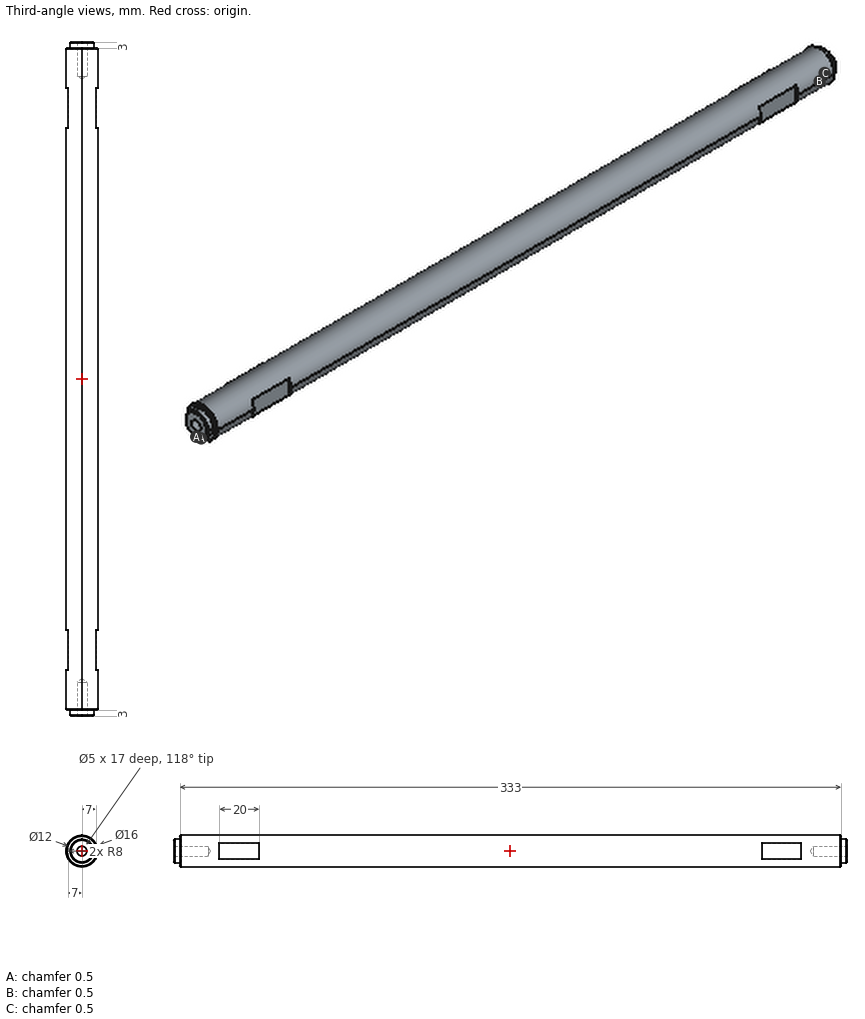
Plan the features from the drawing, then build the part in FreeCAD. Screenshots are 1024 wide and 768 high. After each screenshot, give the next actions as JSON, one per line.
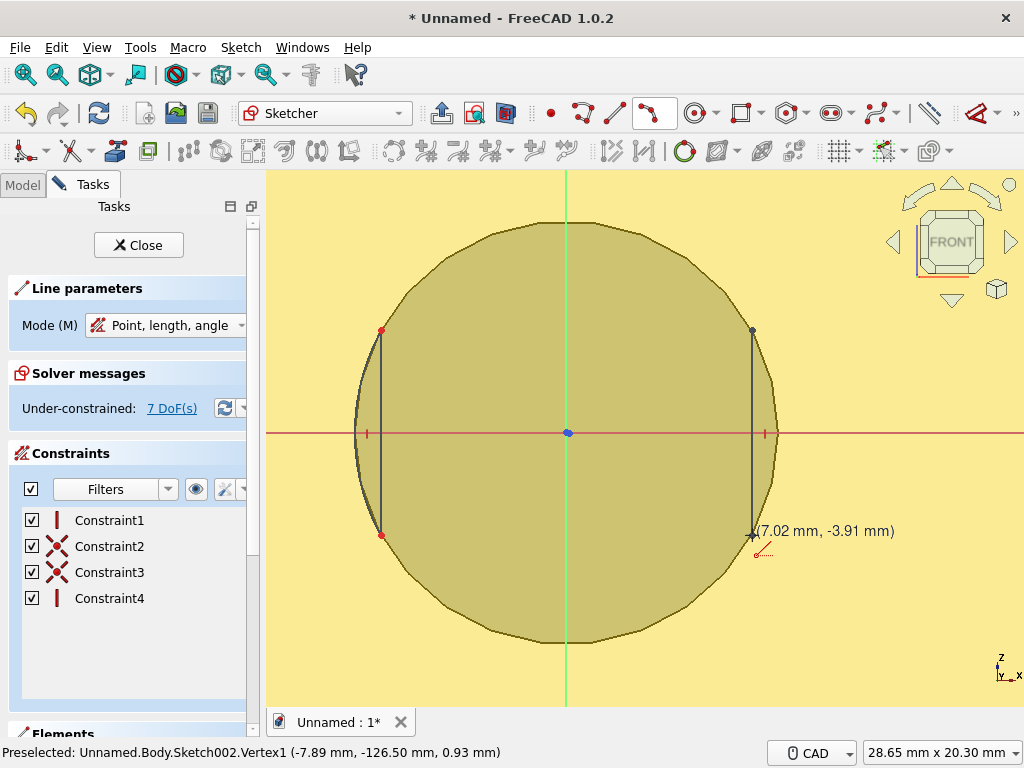
{"action": "key", "text": "g 3 a"}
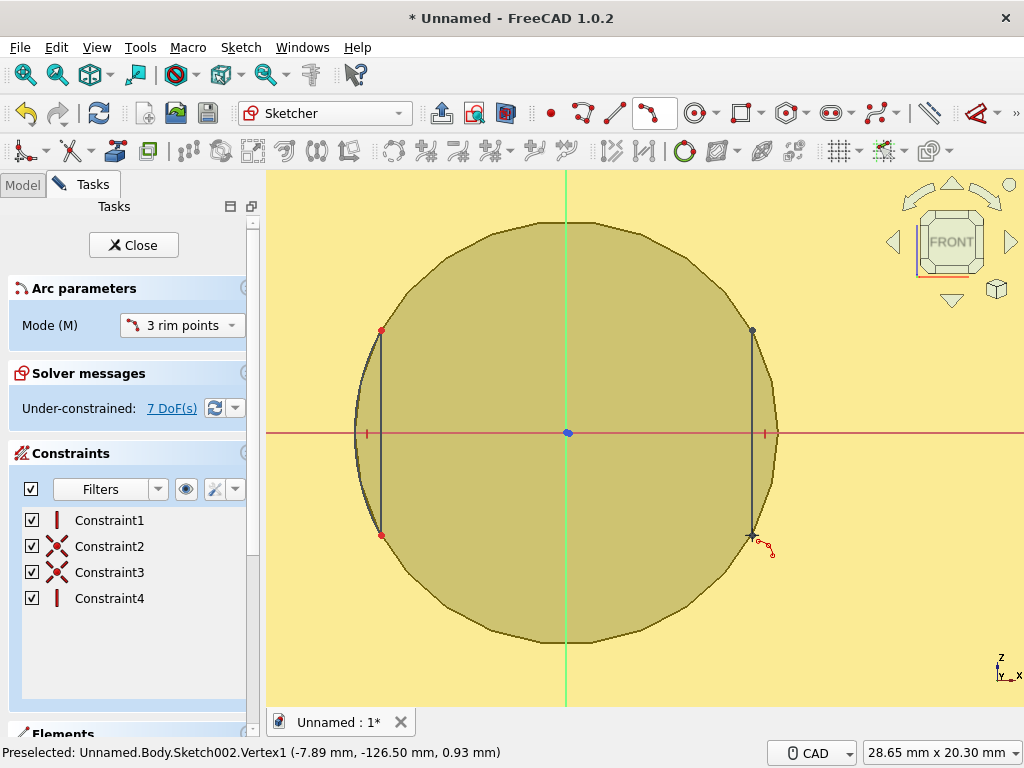
{"action": "left_click", "coordinate": [752, 536]}
{"action": "left_click", "coordinate": [752, 331]}
{"action": "left_click", "coordinate": [777, 454]}
{"action": "key", "text": "Escape"}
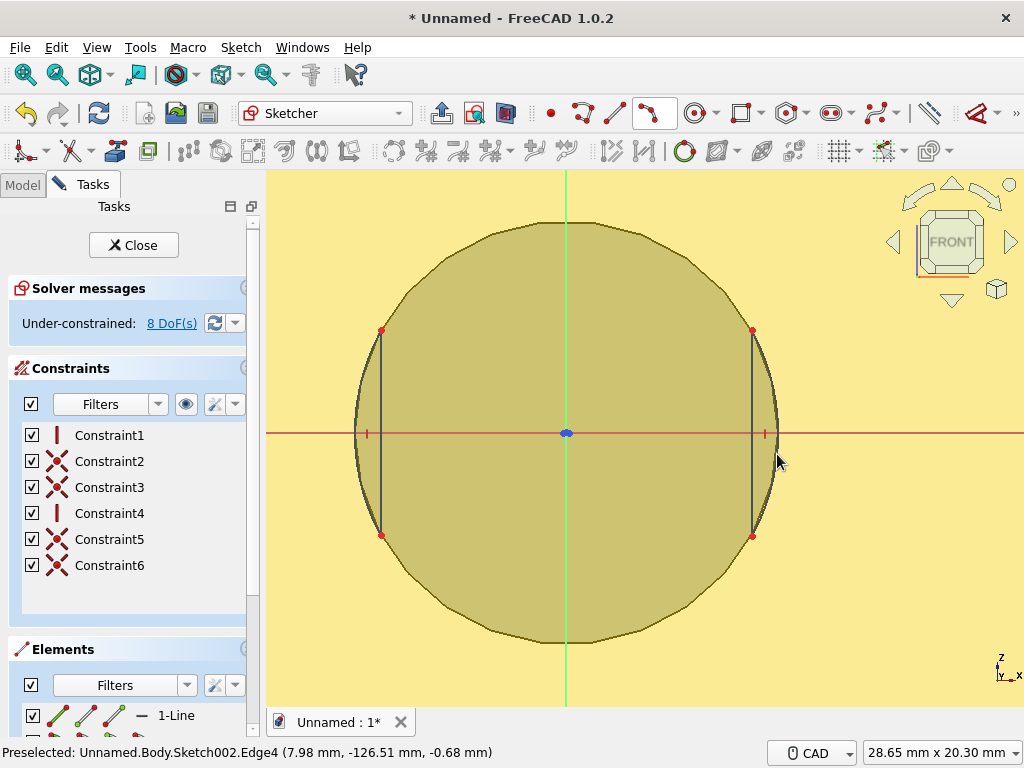
{"action": "left_click", "coordinate": [359, 391]}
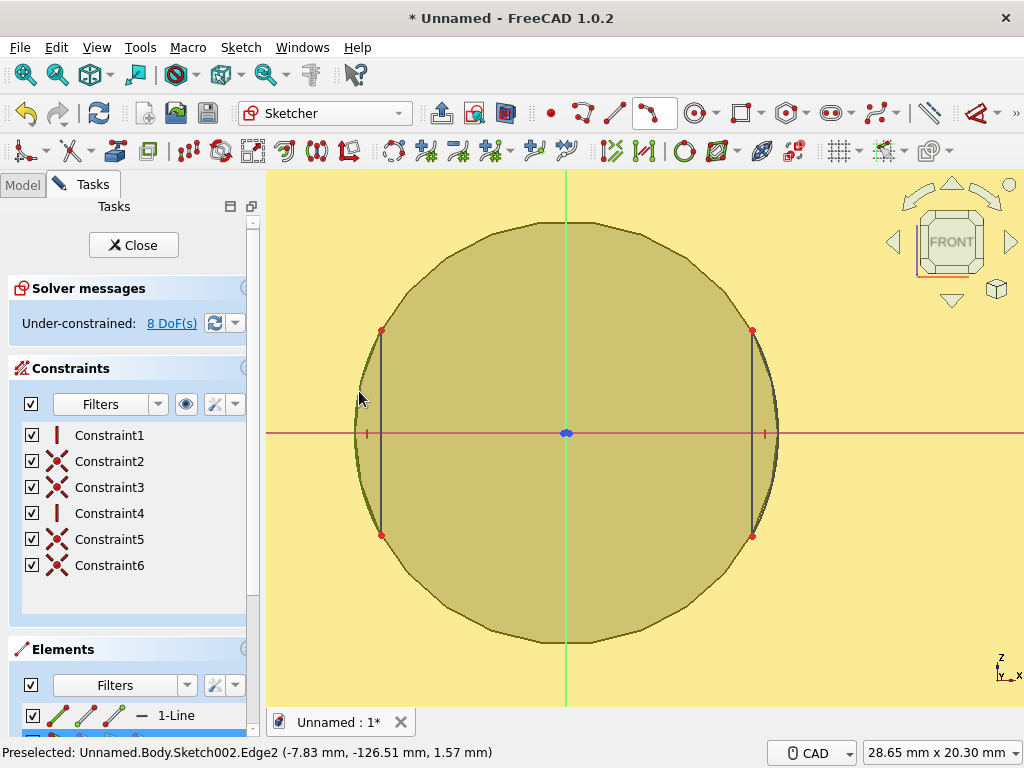
{"action": "left_click", "coordinate": [774, 476]}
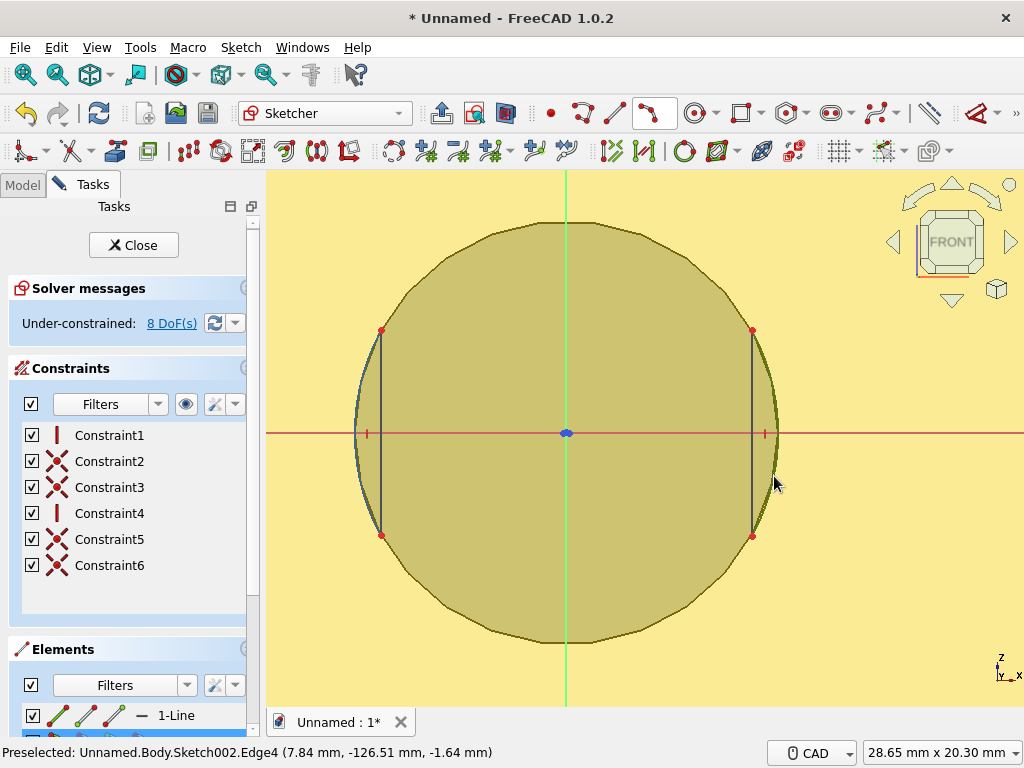
{"action": "key", "text": "c"}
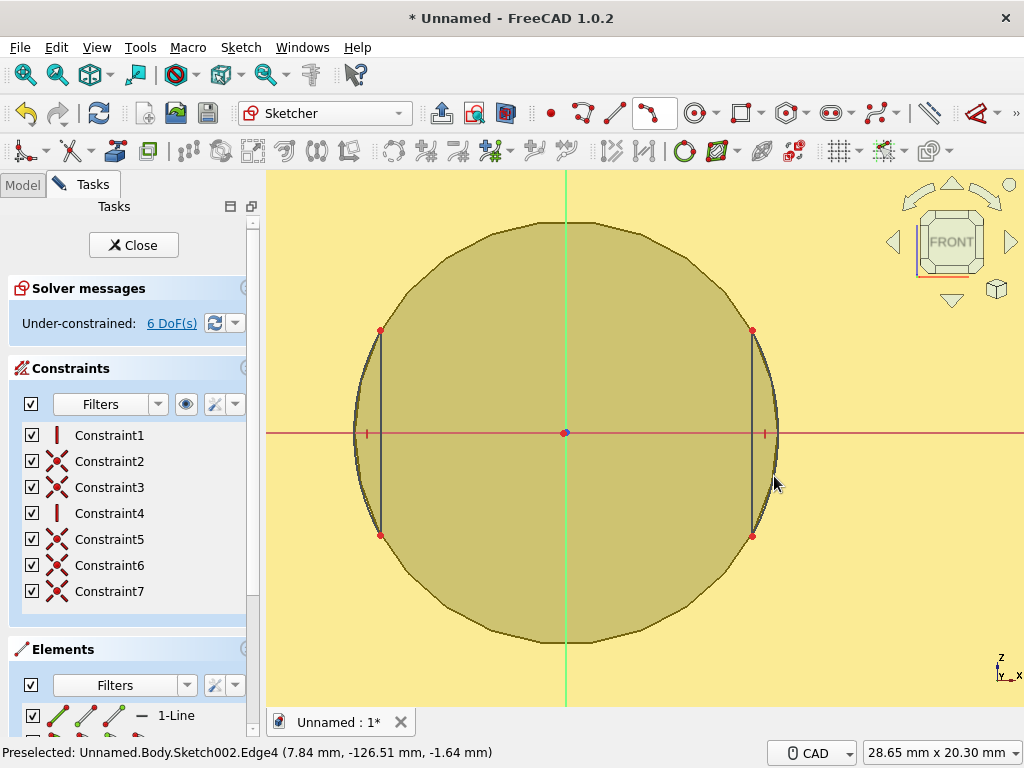
{"action": "left_click_drag", "start_coordinate": [554, 423], "coordinate": [576, 444]}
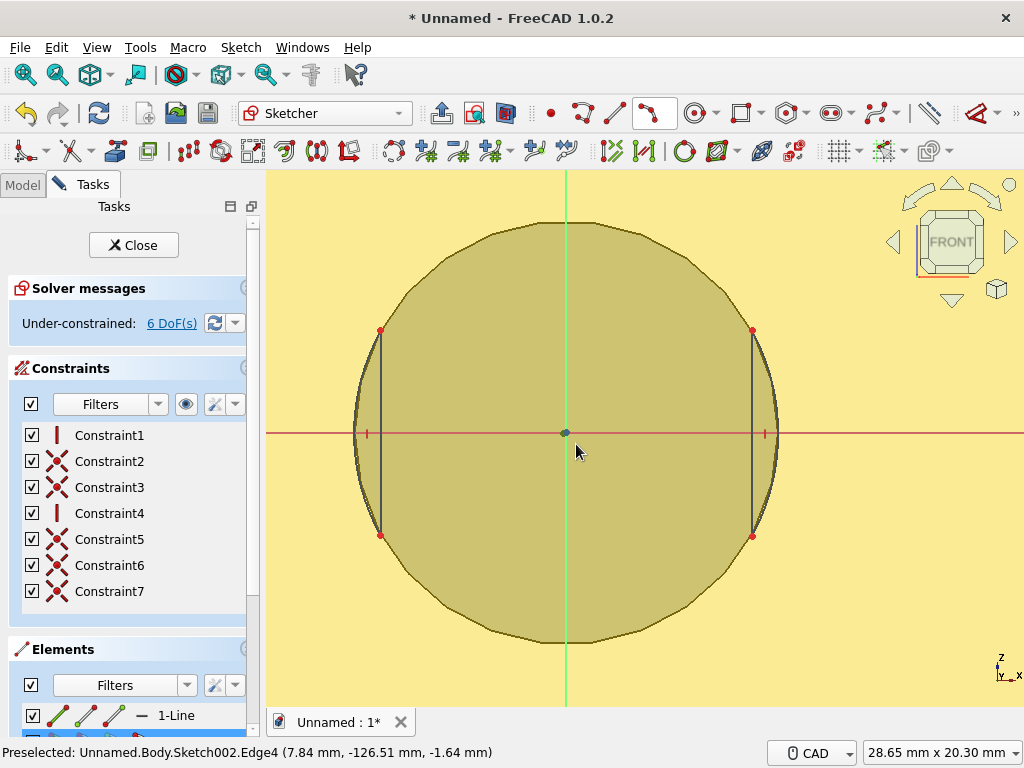
{"action": "key", "text": "c"}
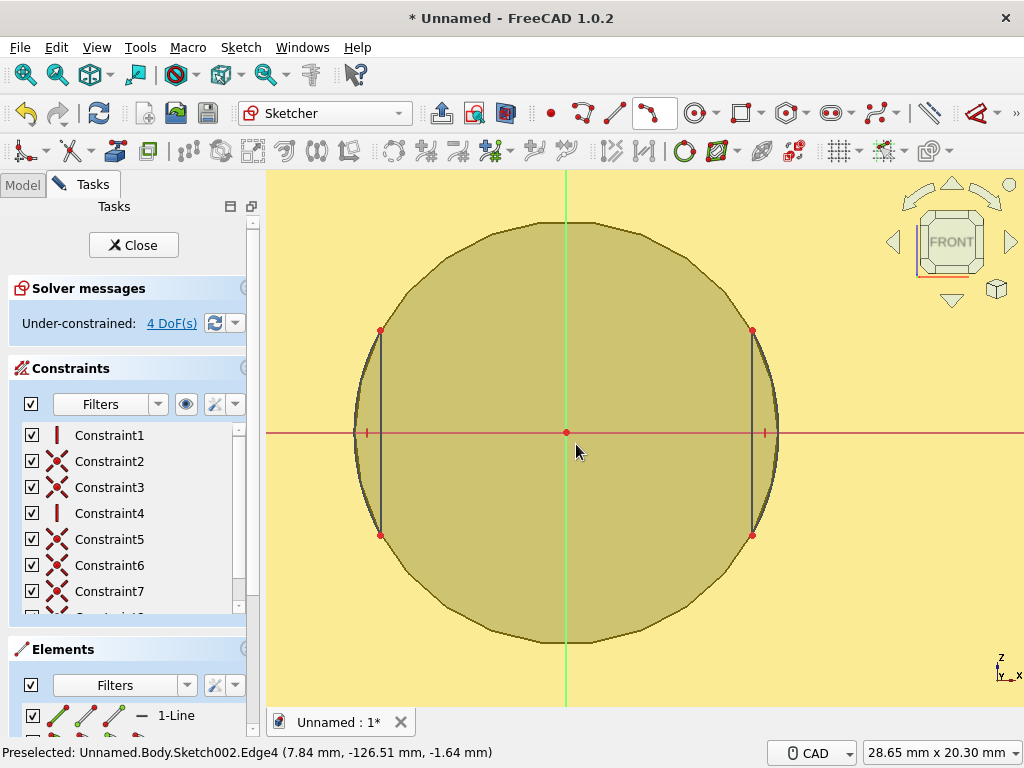
{"action": "left_click", "coordinate": [359, 390]}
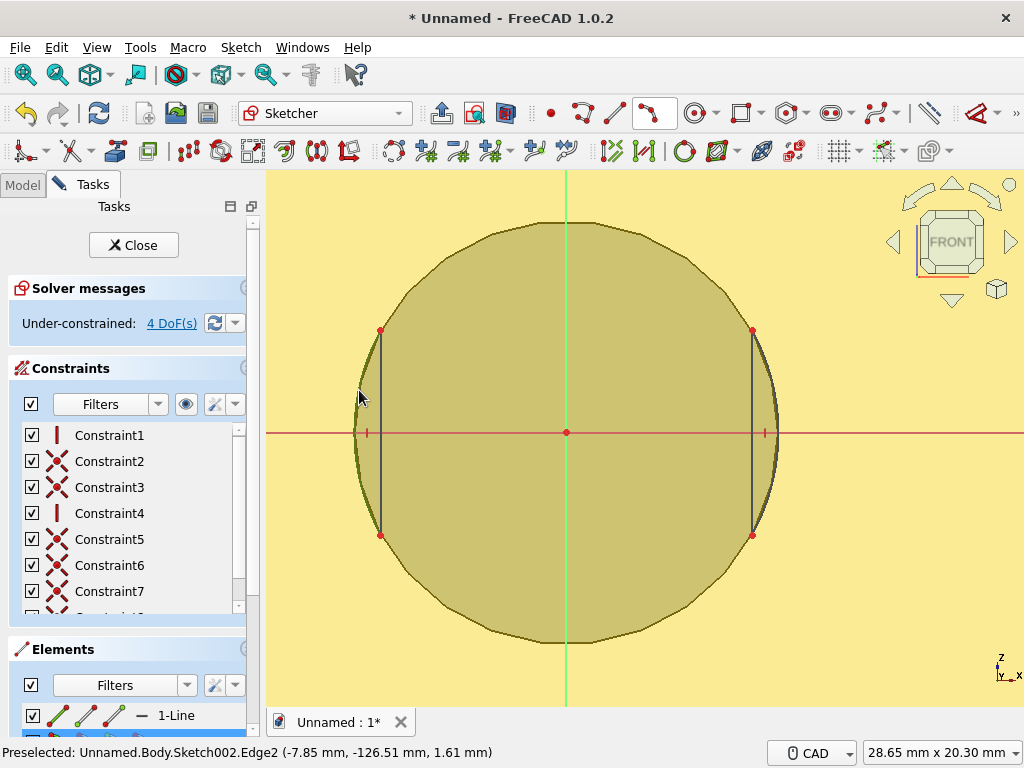
{"action": "left_click", "coordinate": [774, 475]}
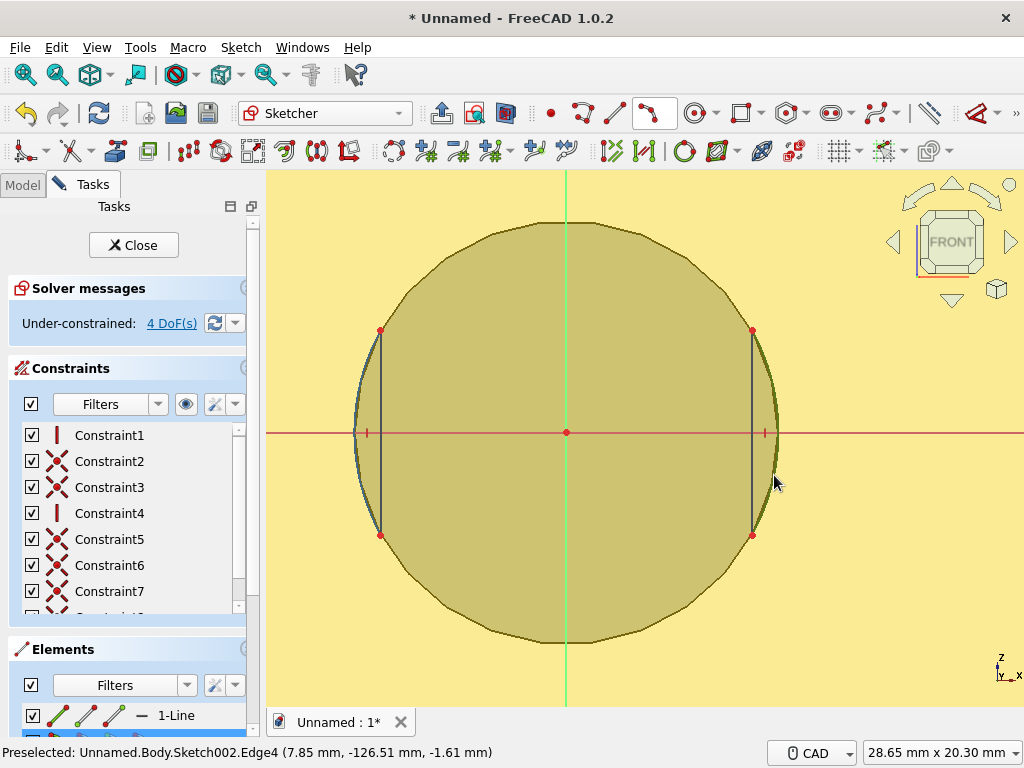
{"action": "key", "text": "e"}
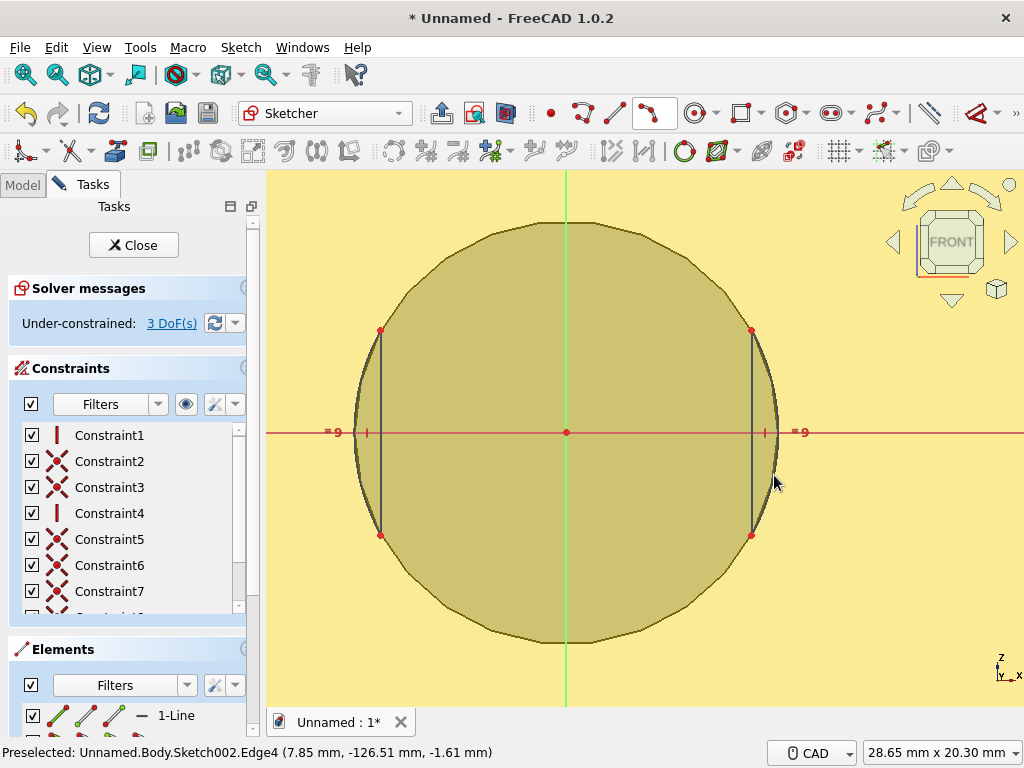
{"action": "key", "text": "d"}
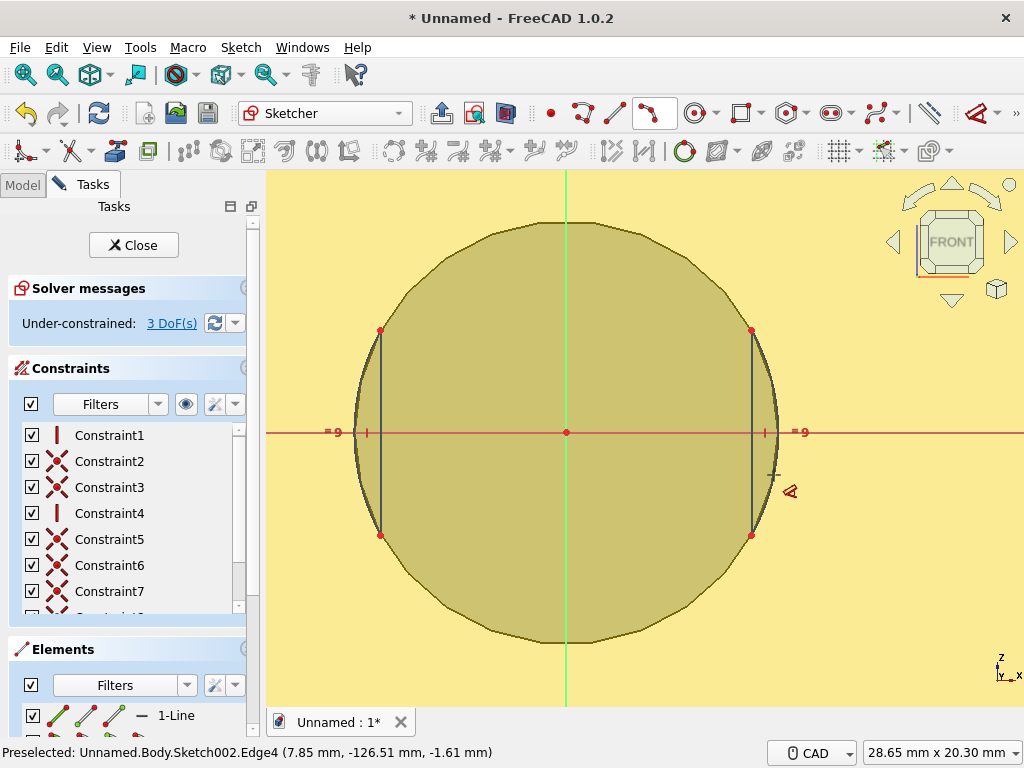
{"action": "left_click", "coordinate": [359, 390]}
{"action": "left_click", "coordinate": [328, 384]}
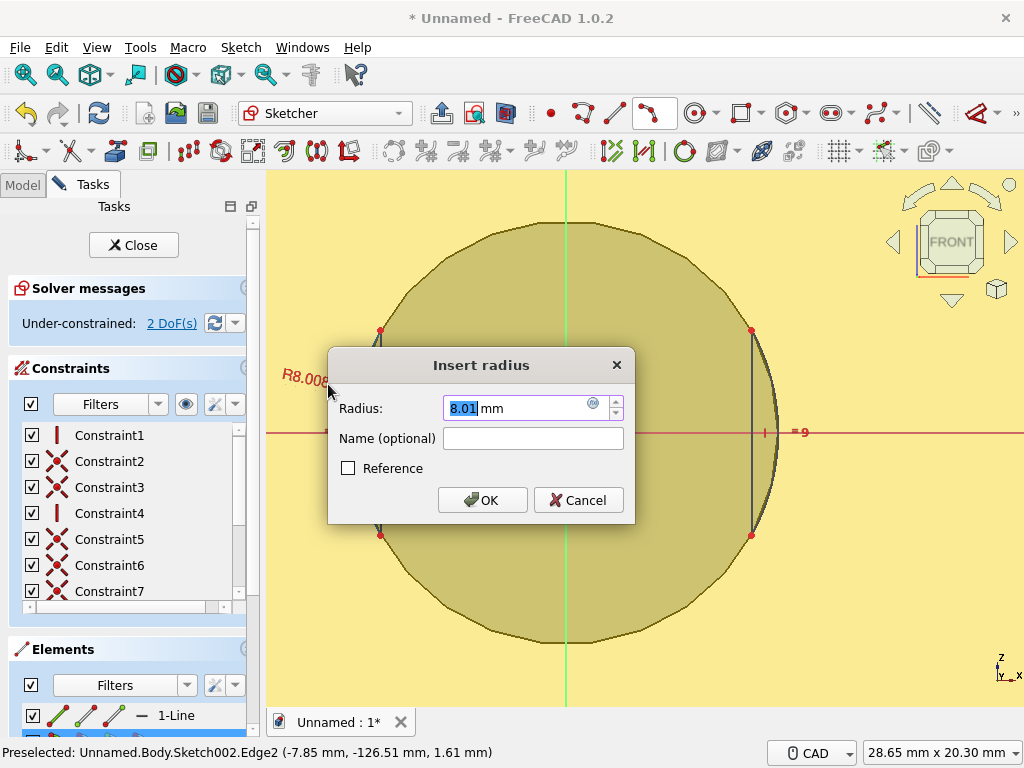
{"action": "type", "text": "8"}
{"action": "key", "text": "Return"}